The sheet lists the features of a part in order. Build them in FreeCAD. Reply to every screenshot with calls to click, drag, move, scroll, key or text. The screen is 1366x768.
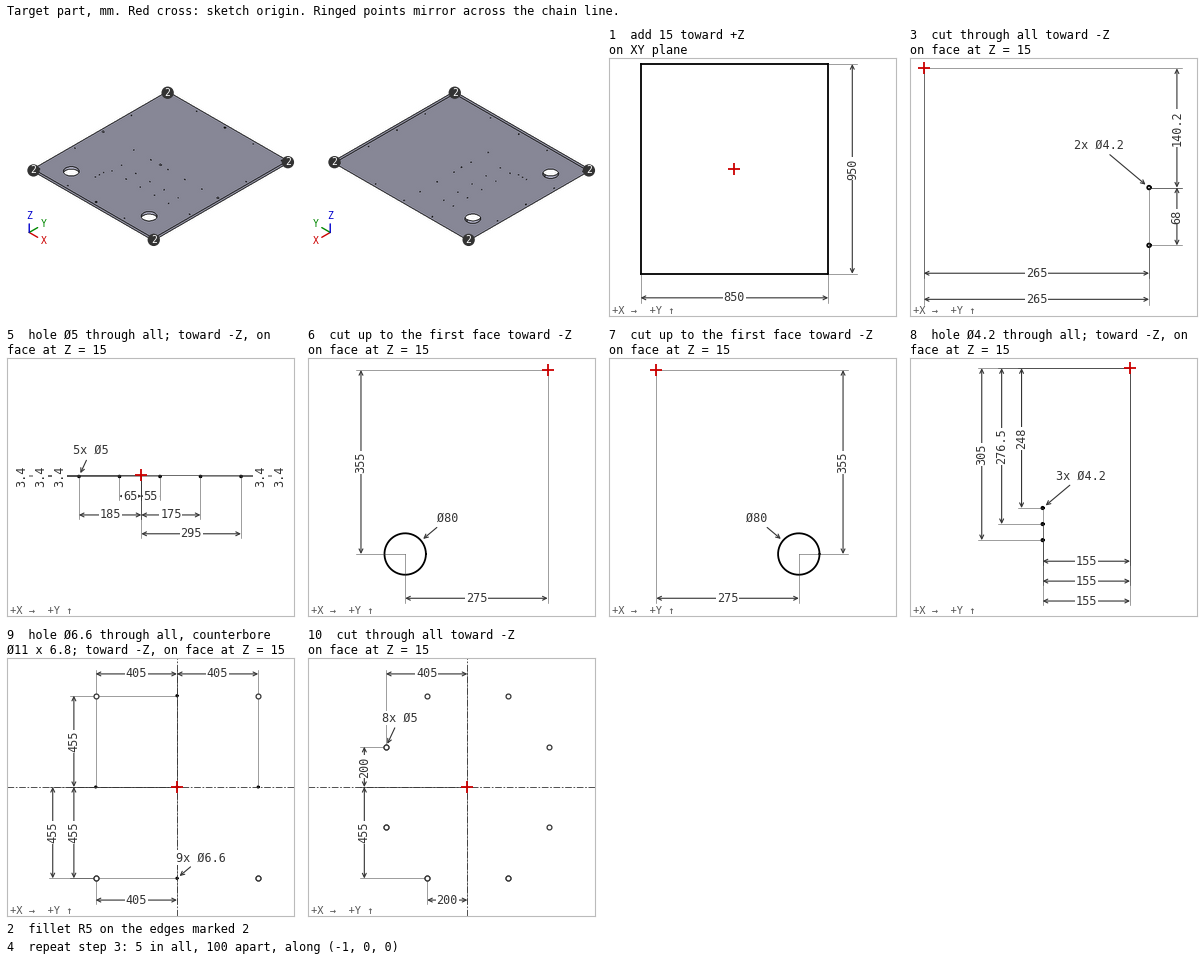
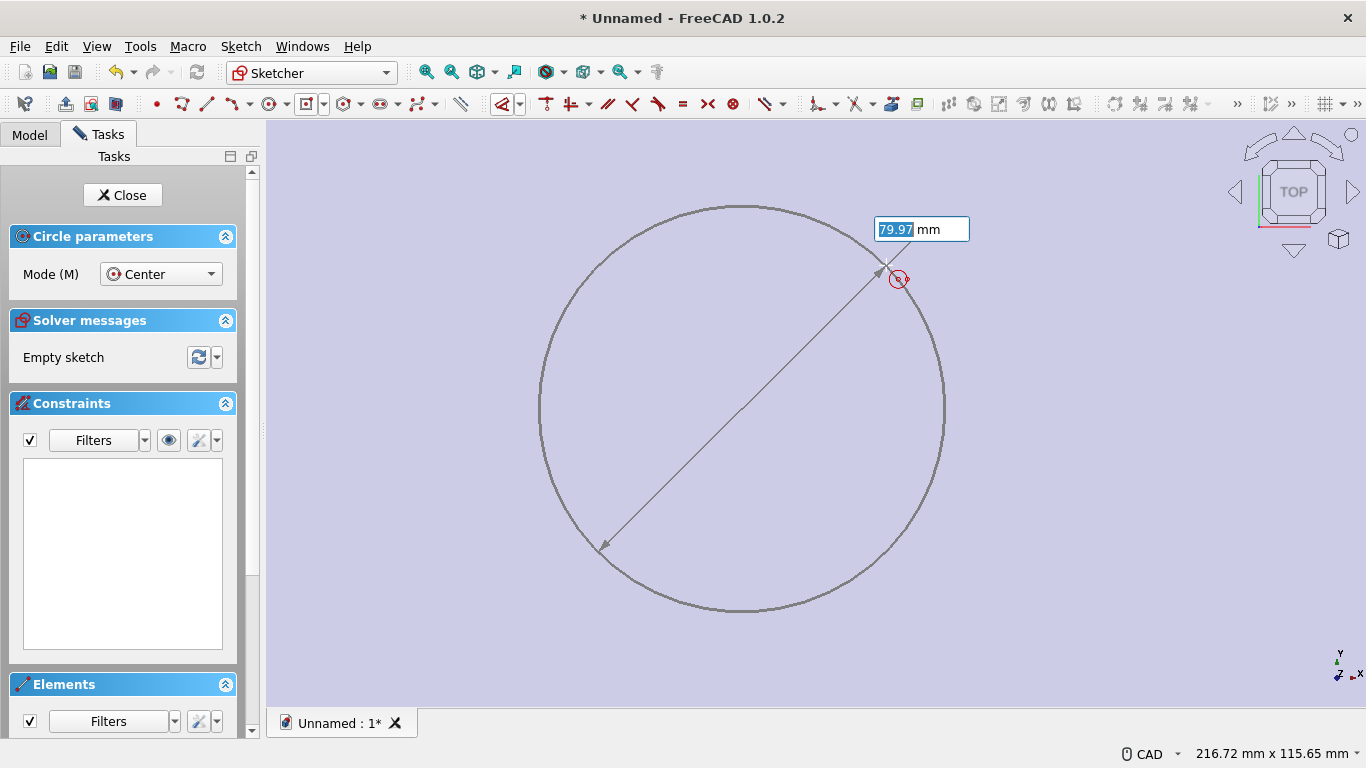
text(80)
key(Return)
key(Escape)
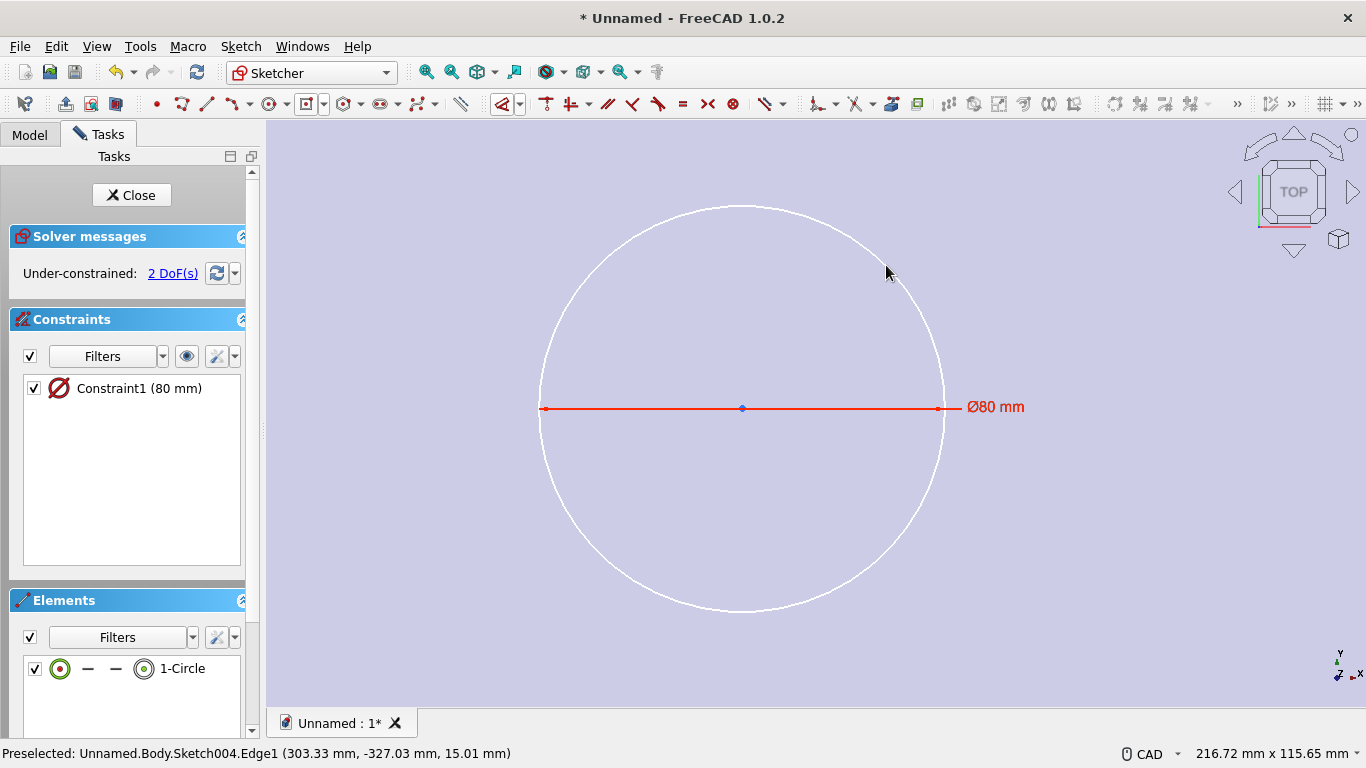
click(742, 409)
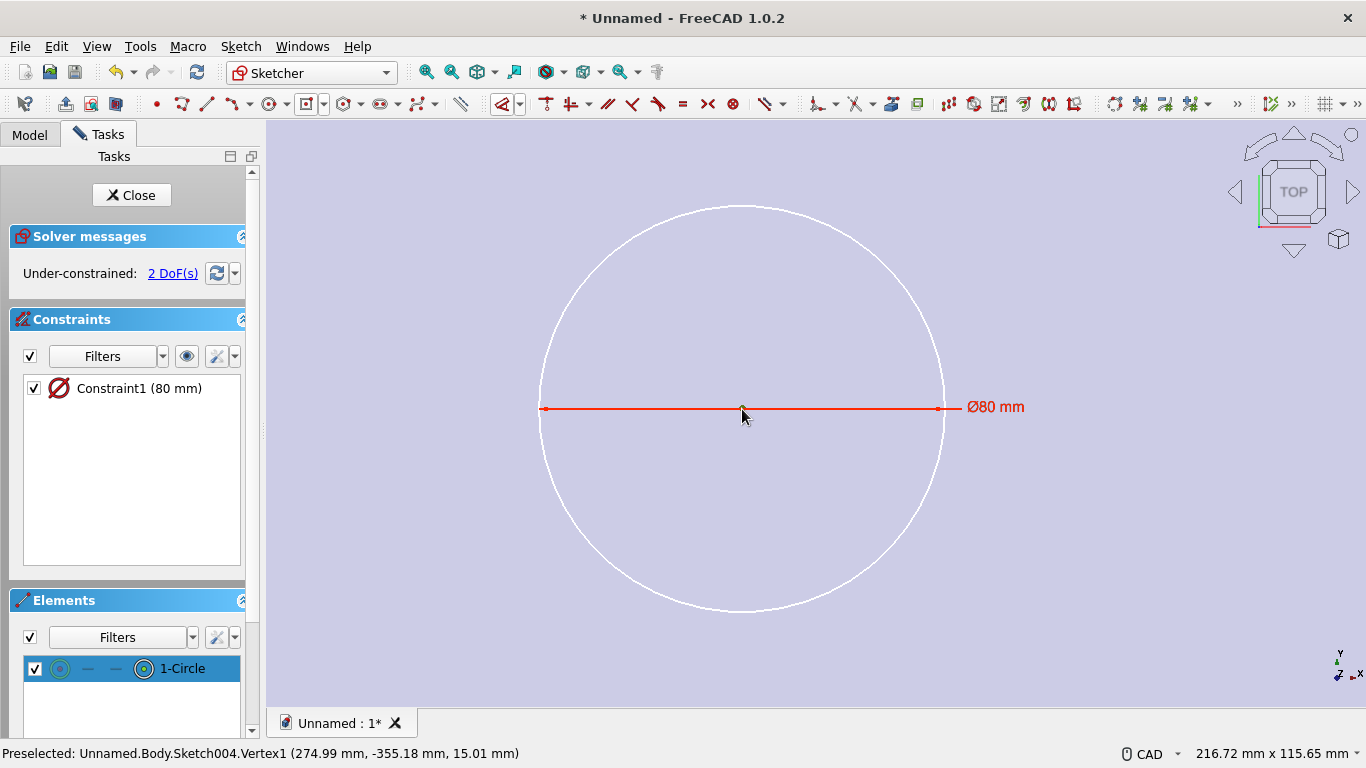
key(l)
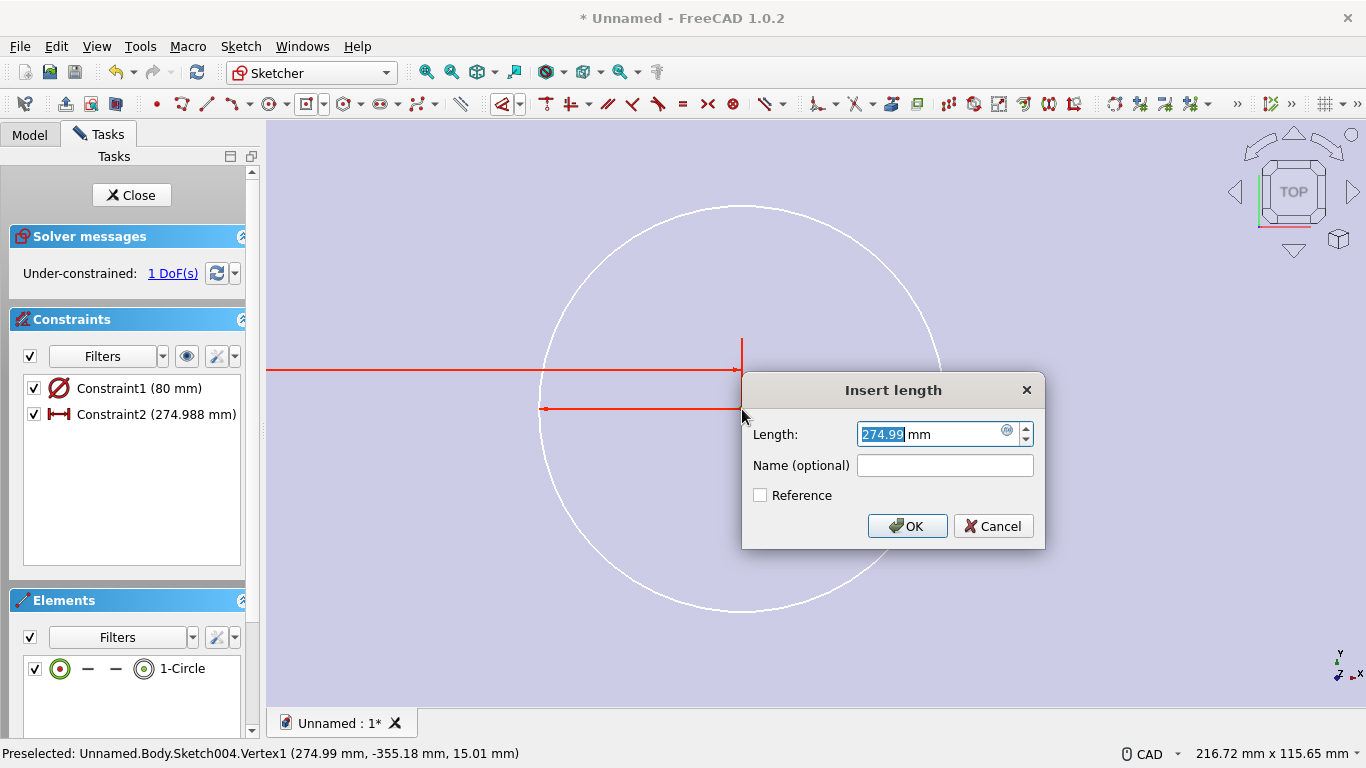
text(275)
key(Return)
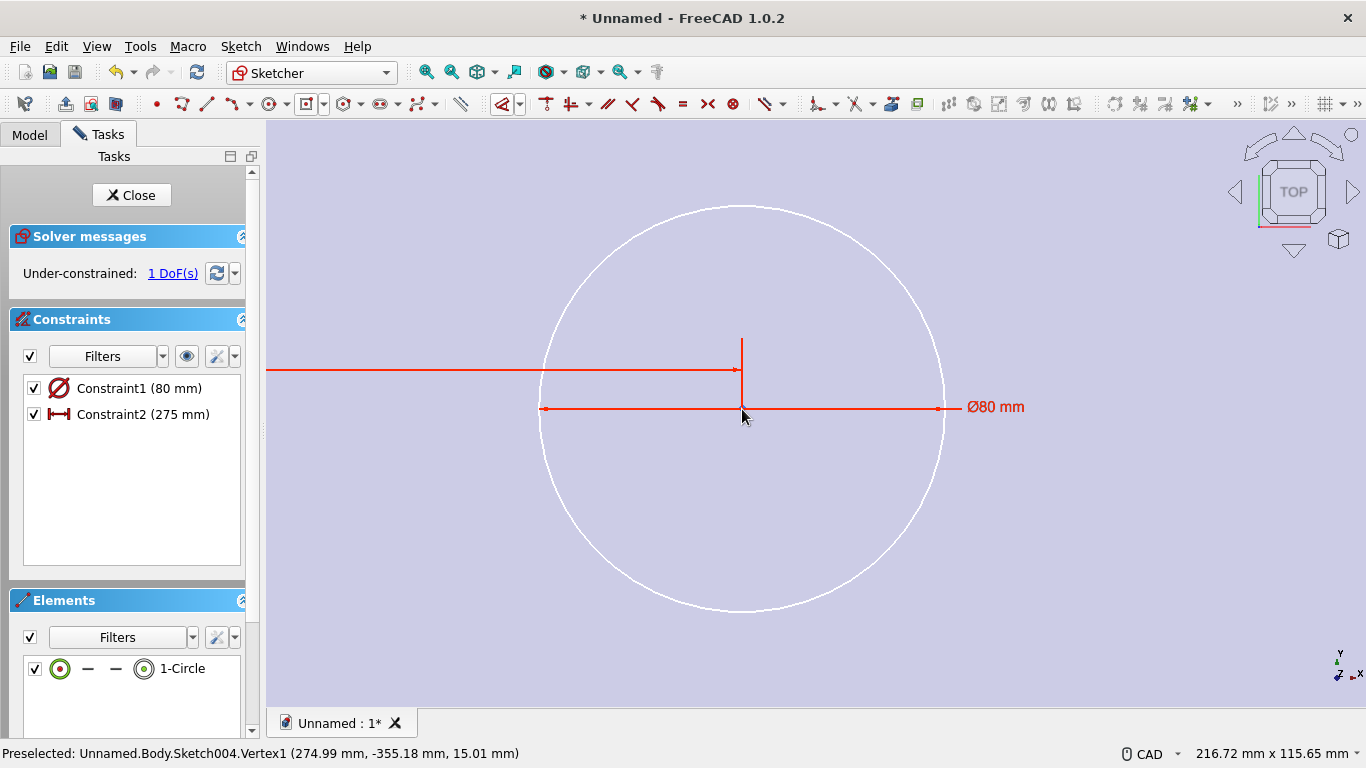
click(742, 409)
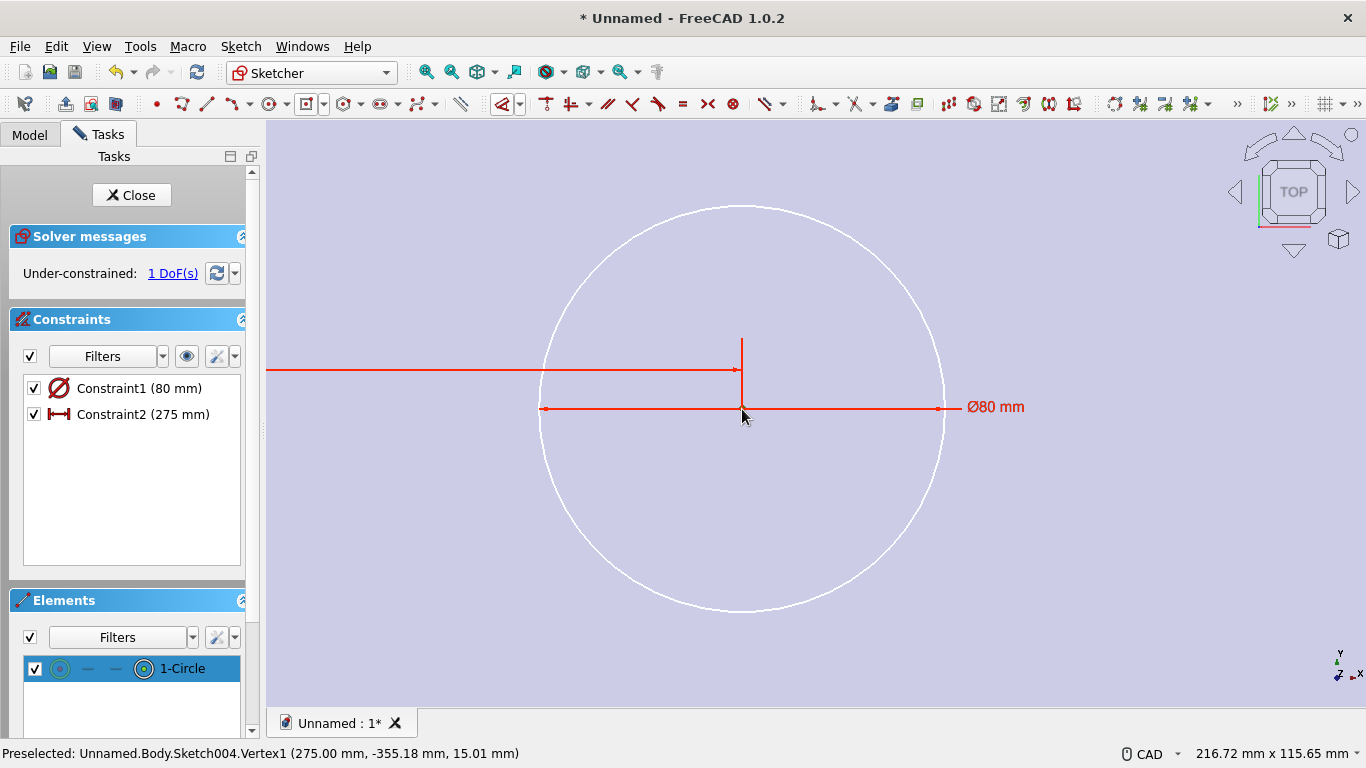
click(520, 104)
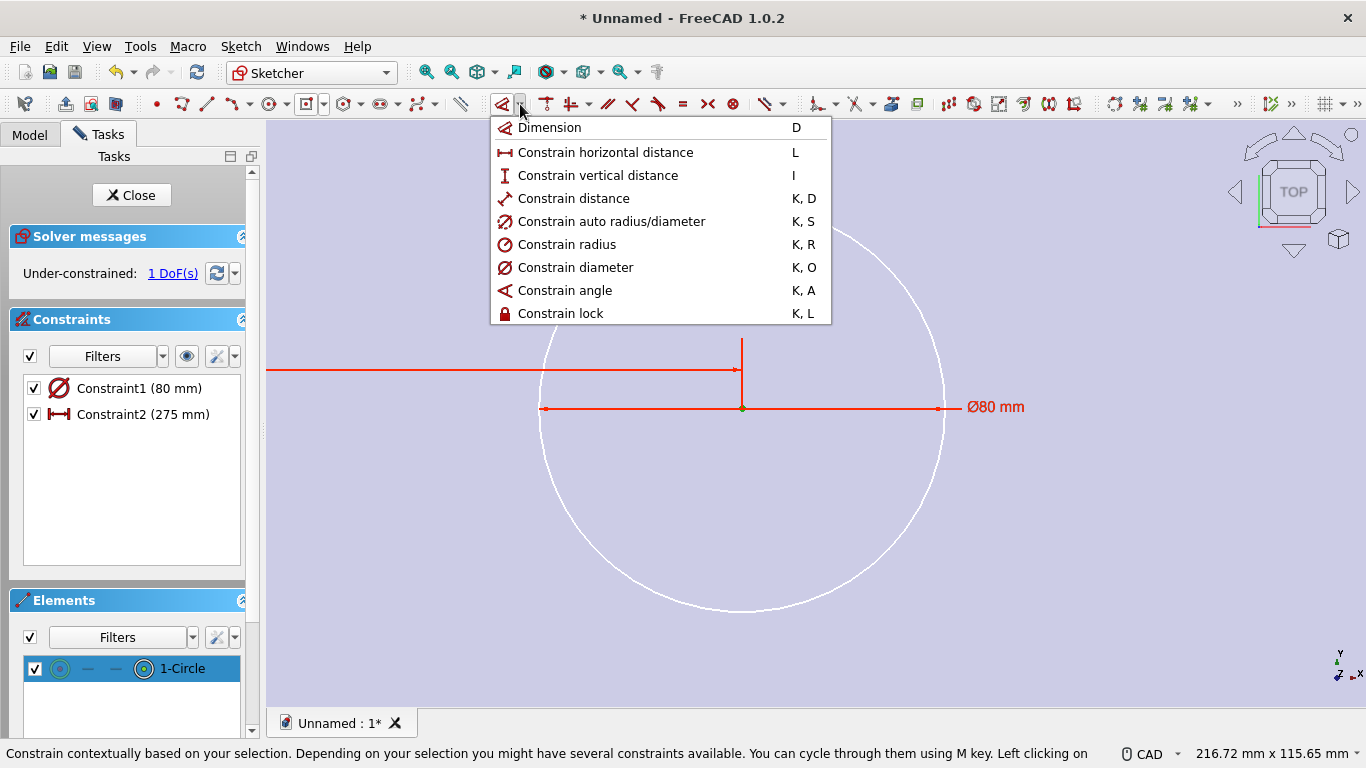
click(661, 176)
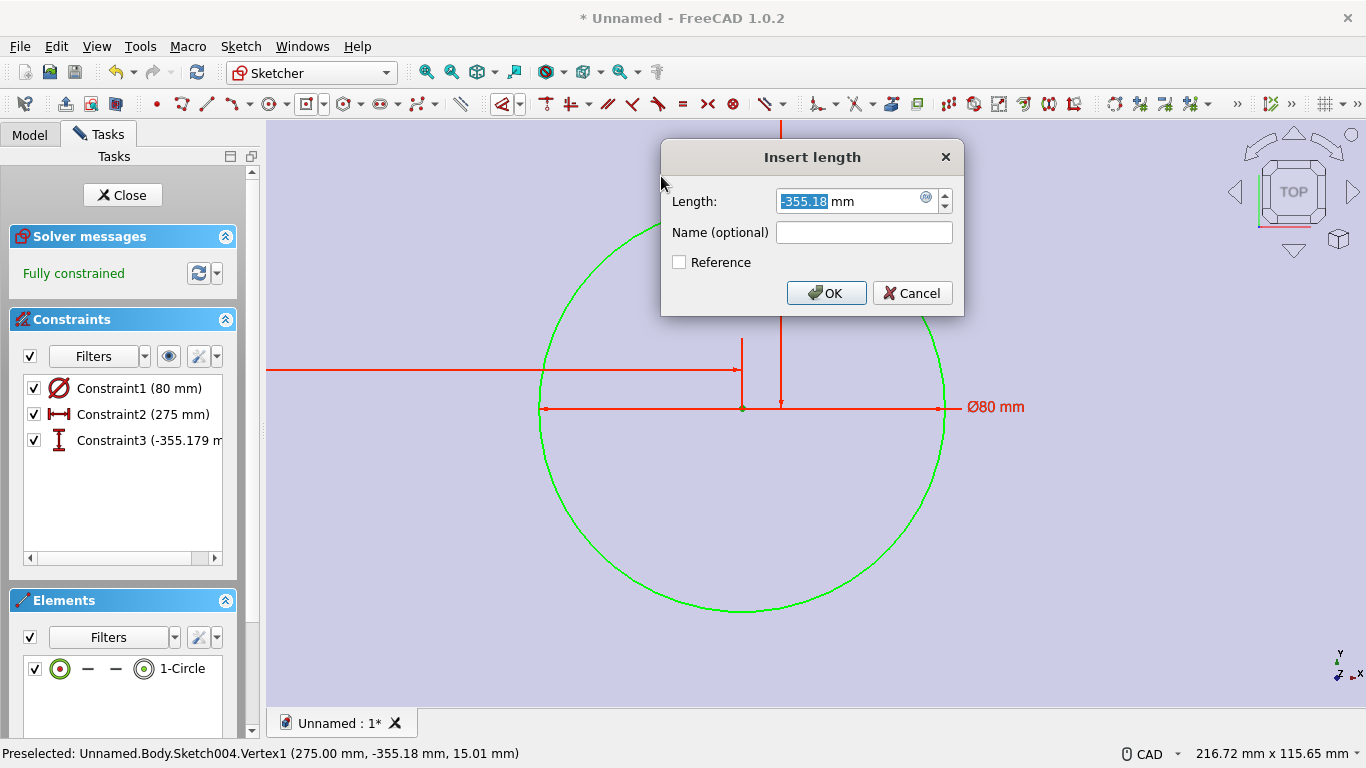
text(-355)
key(Return)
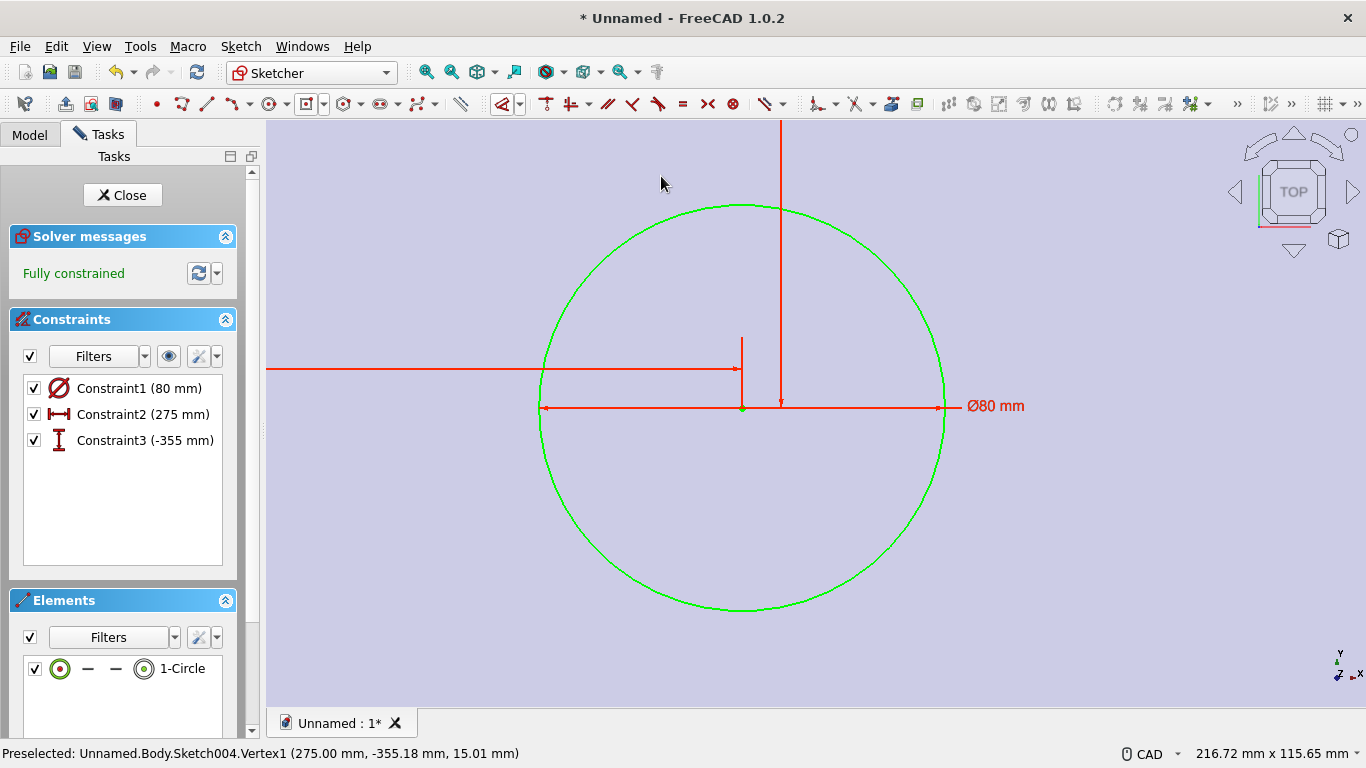
click(123, 195)